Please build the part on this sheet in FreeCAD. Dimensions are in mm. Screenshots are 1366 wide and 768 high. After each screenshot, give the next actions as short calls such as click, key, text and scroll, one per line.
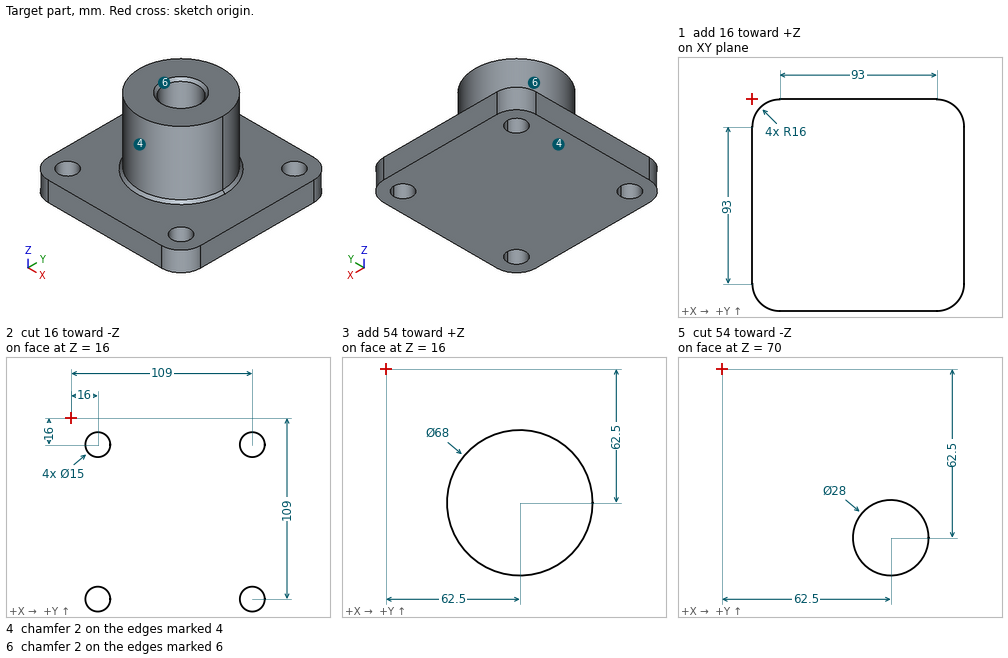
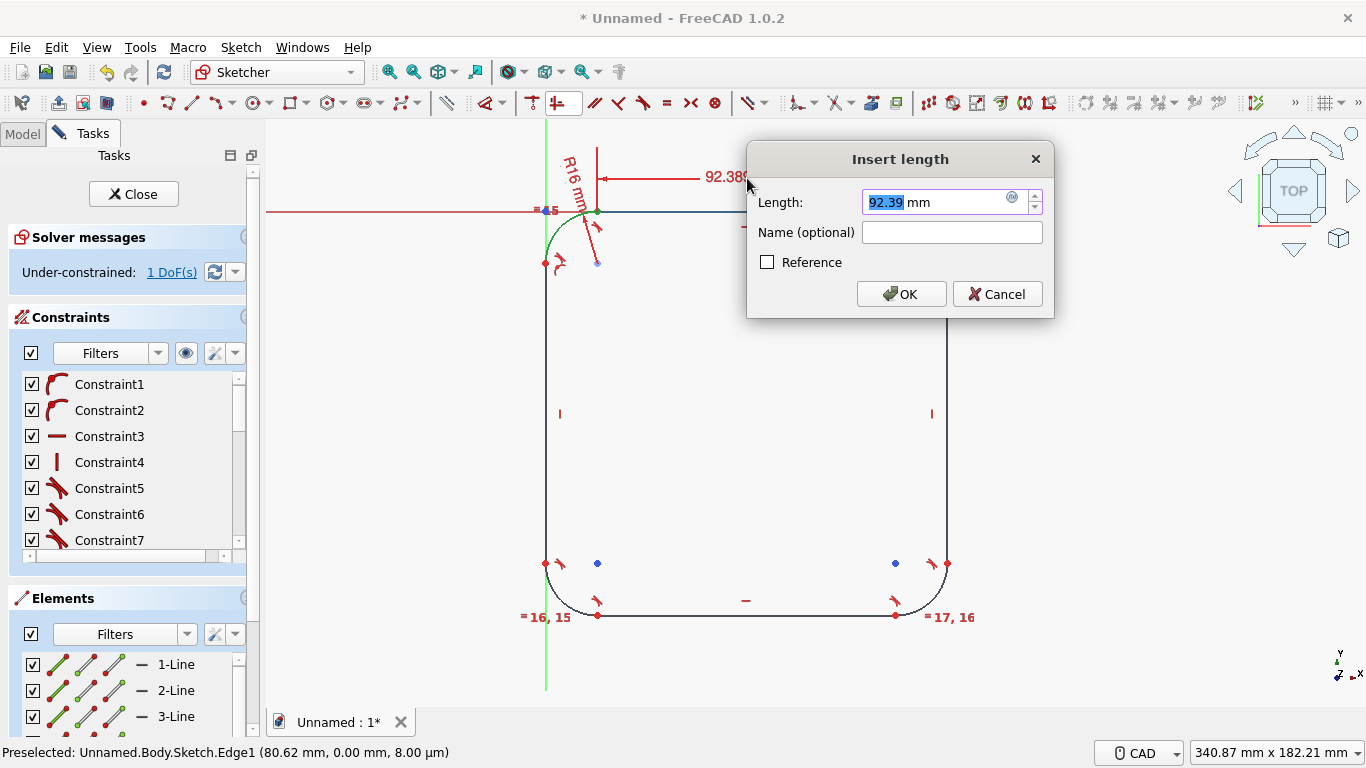
text(93)
key(Return)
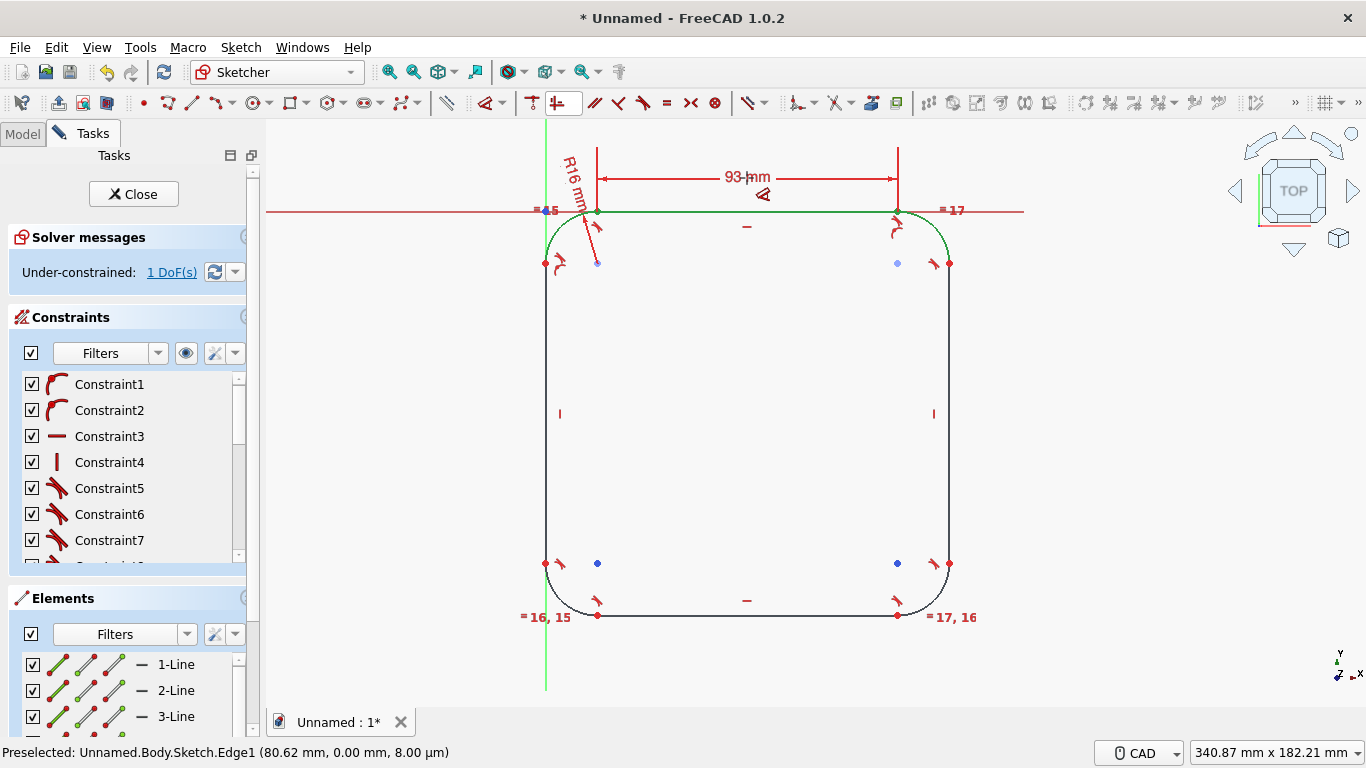
click(546, 353)
click(512, 414)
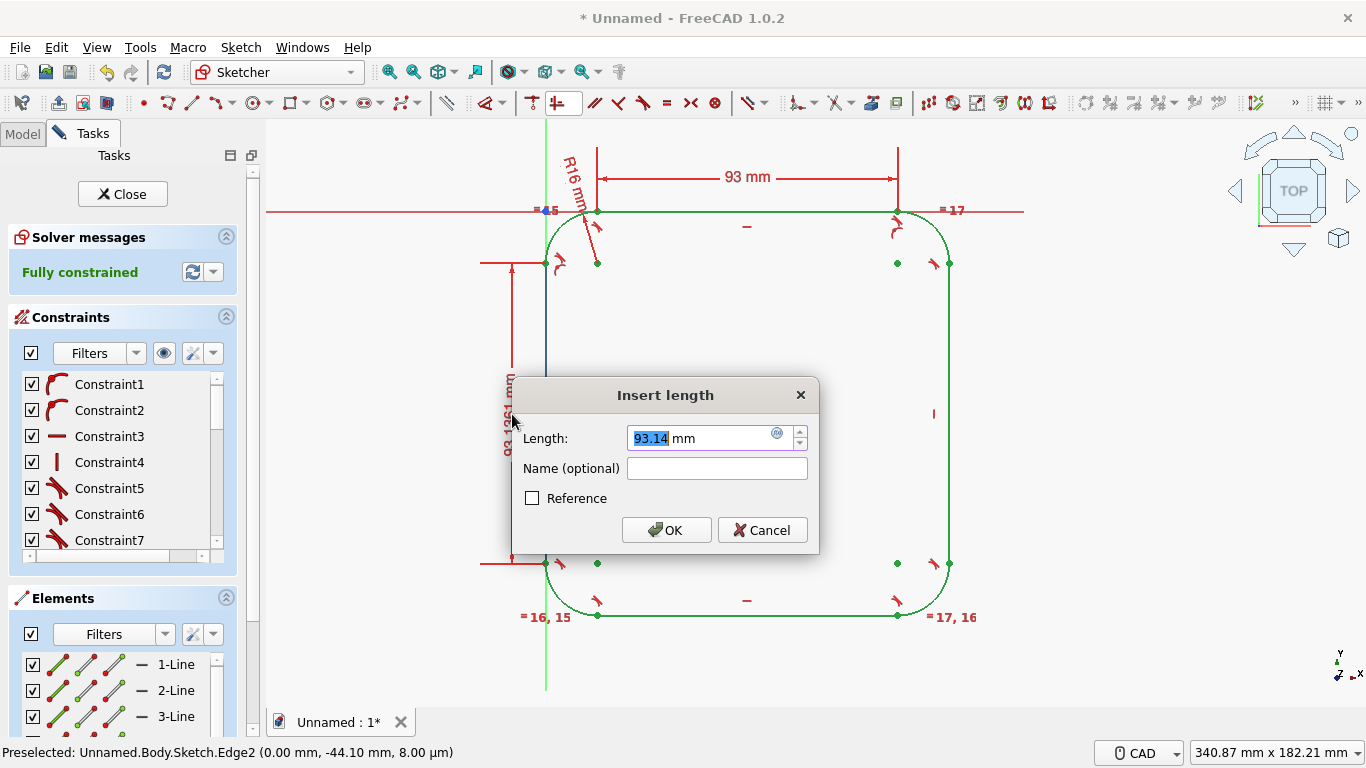
text(93)
key(Return)
key(Escape)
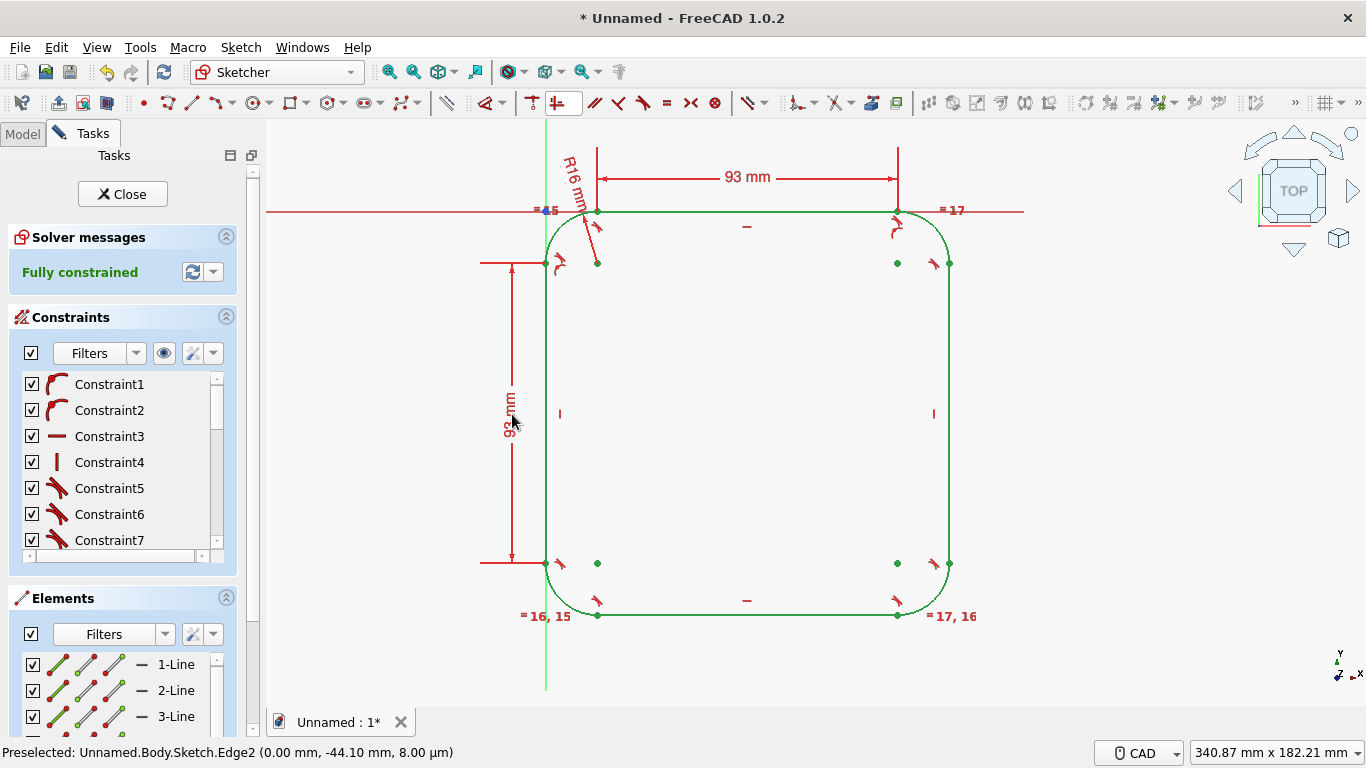
click(123, 194)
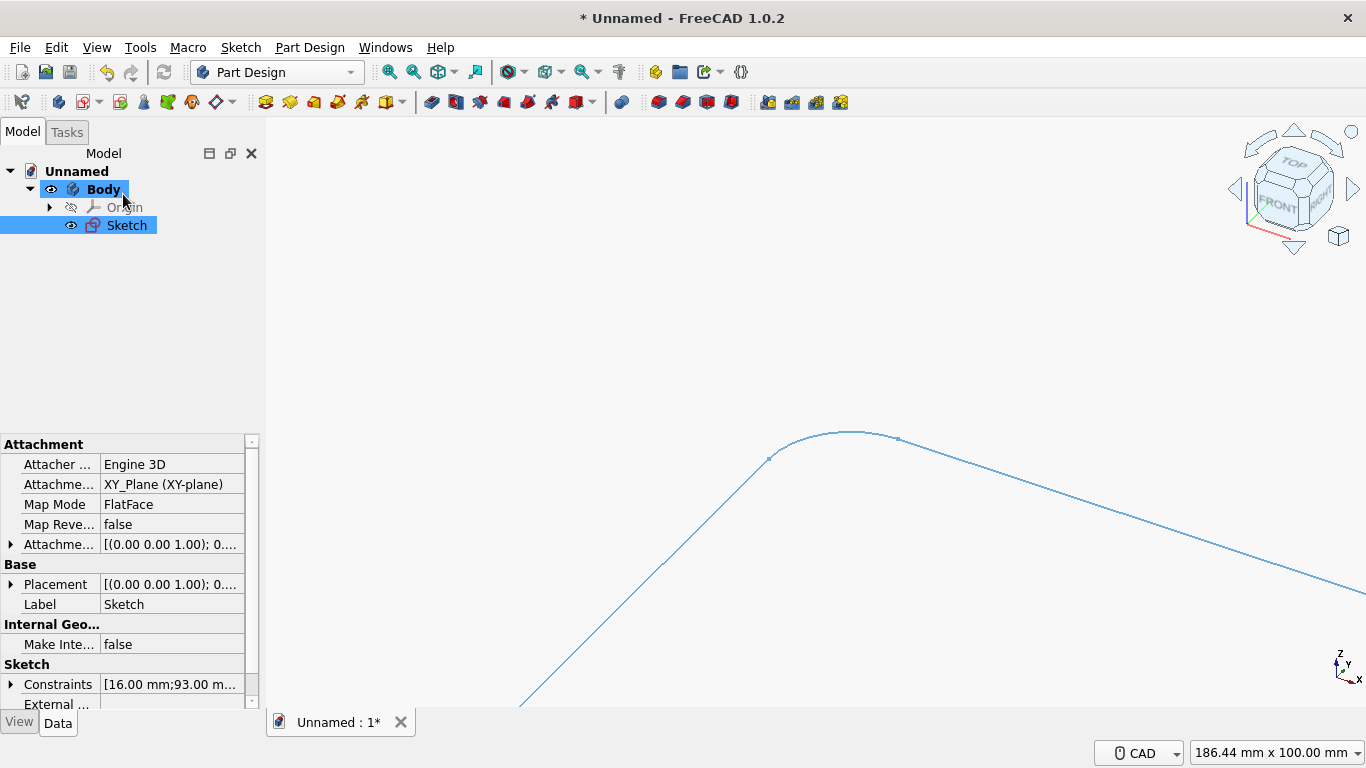
click(266, 102)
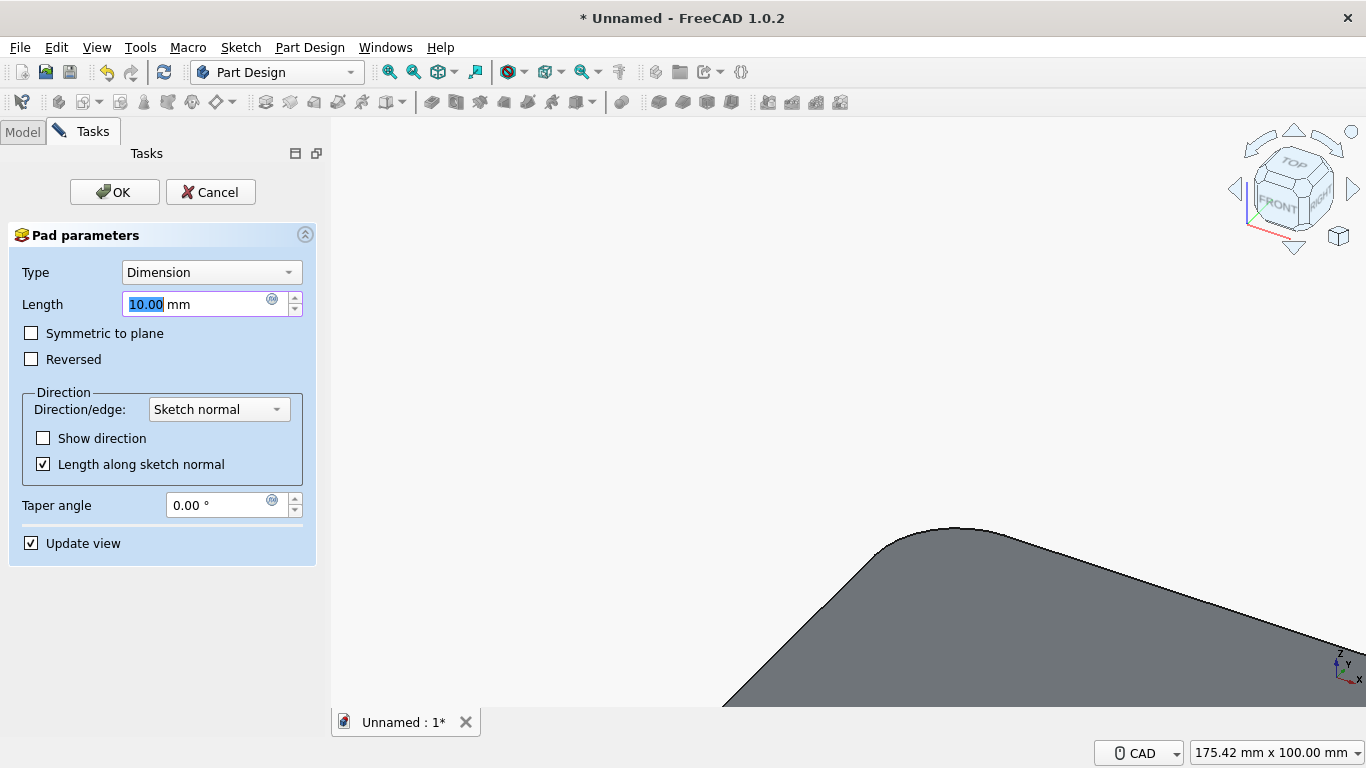
text(16)
key(Tab)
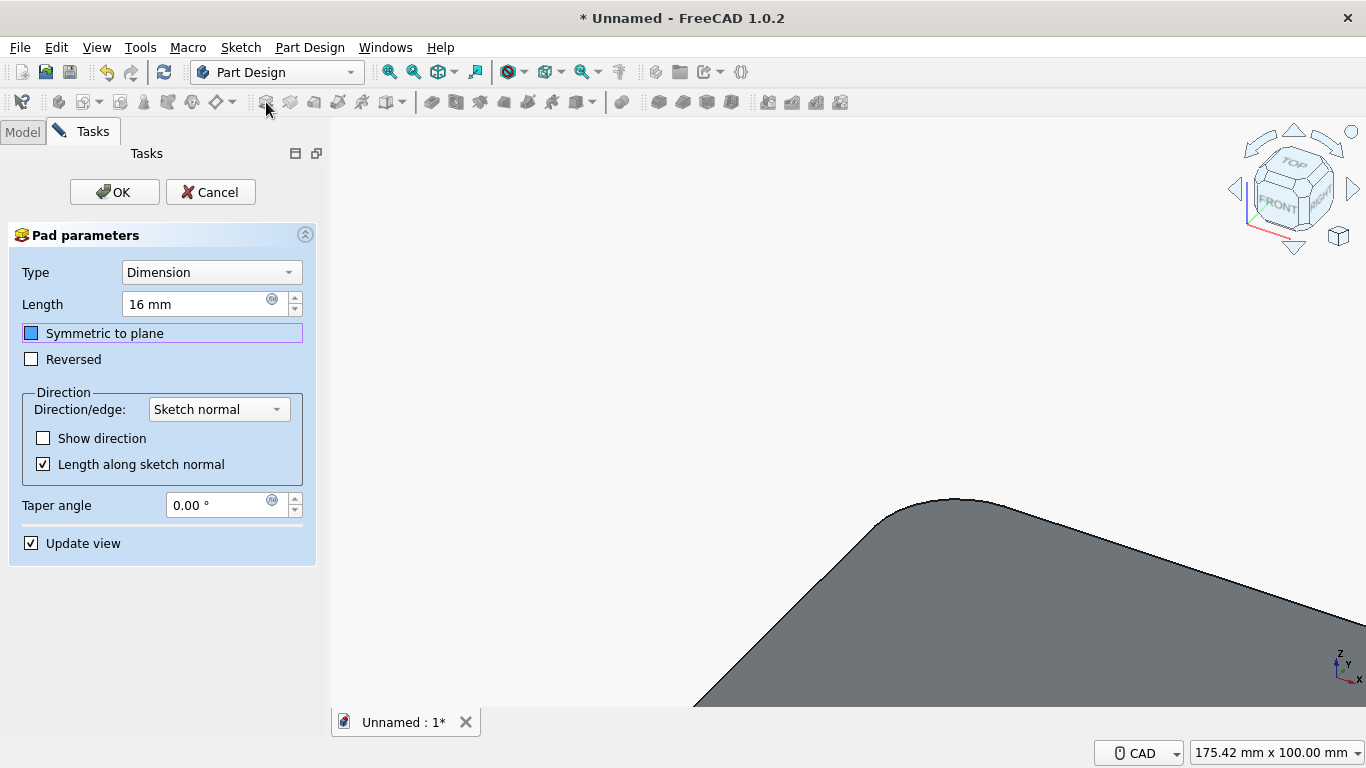
click(115, 192)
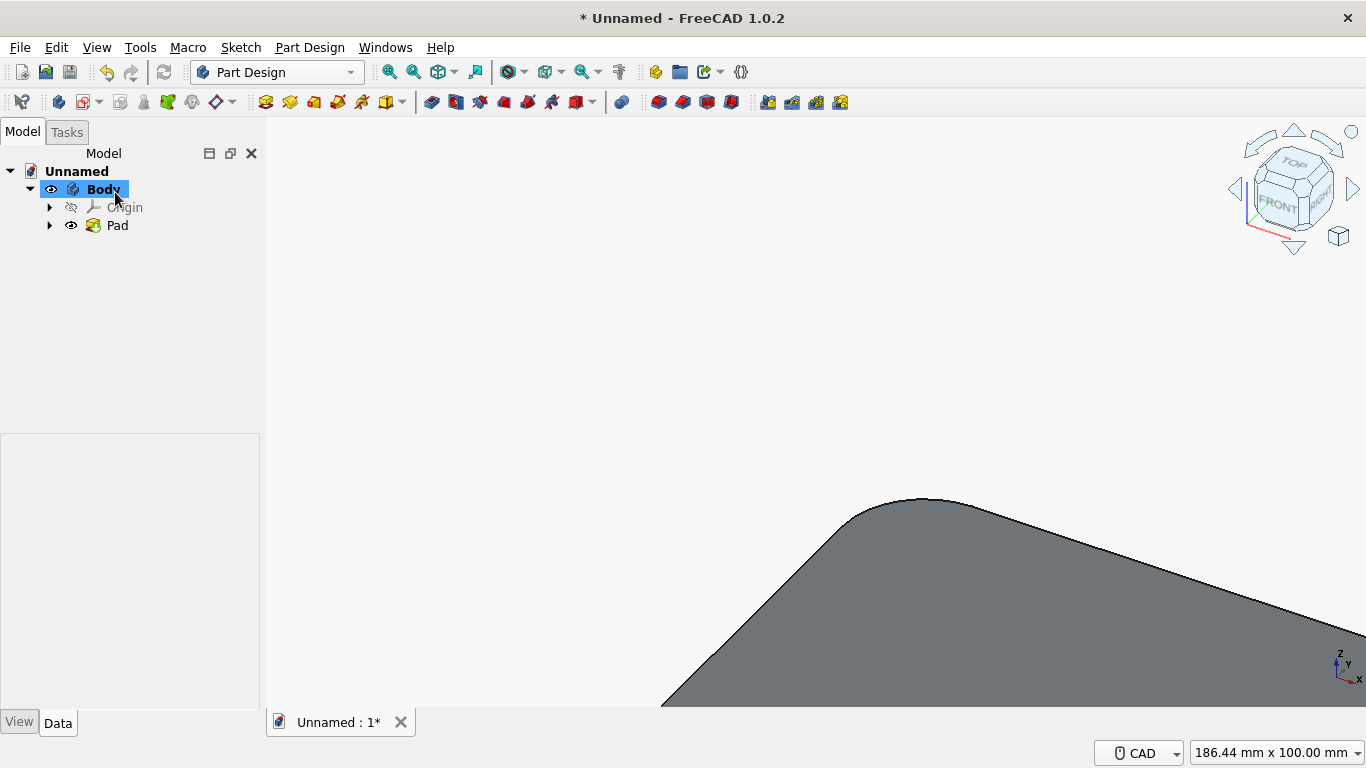
key(v)
key(f)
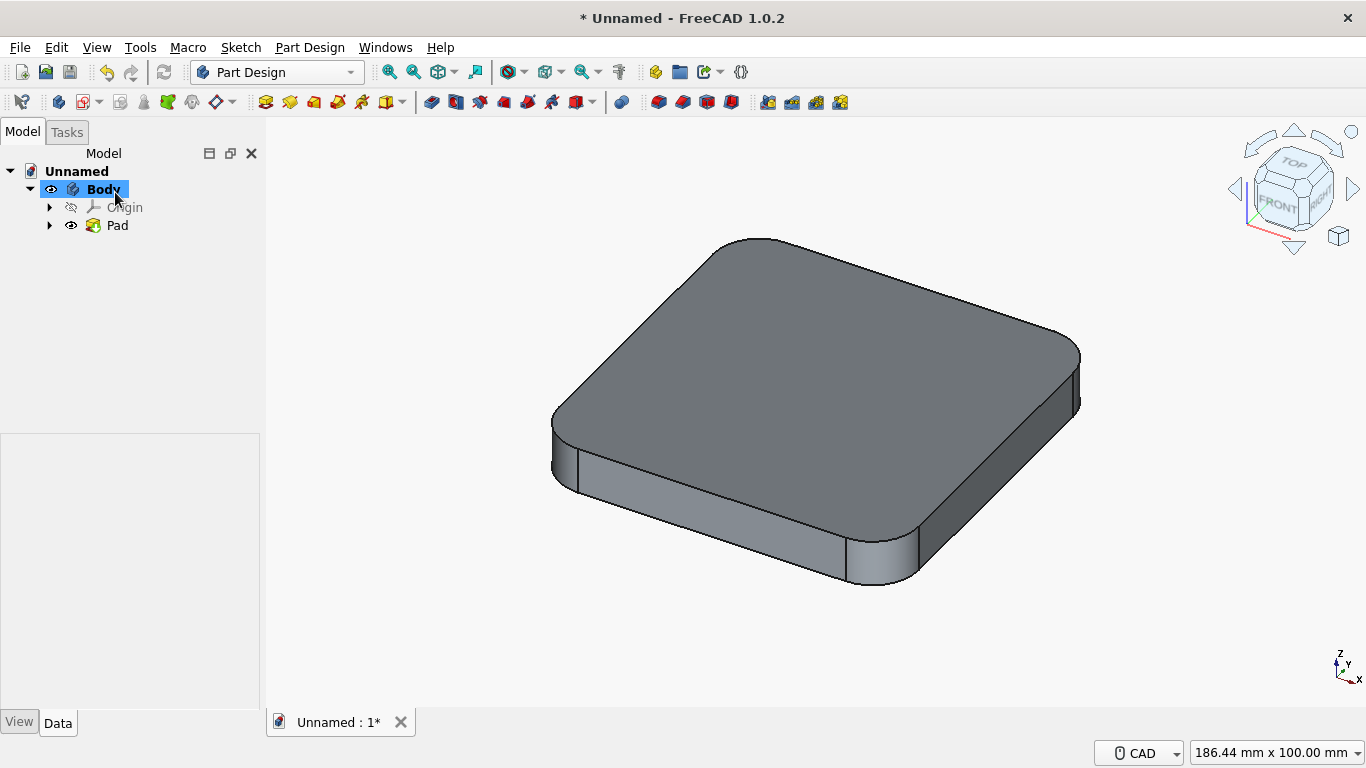
click(816, 389)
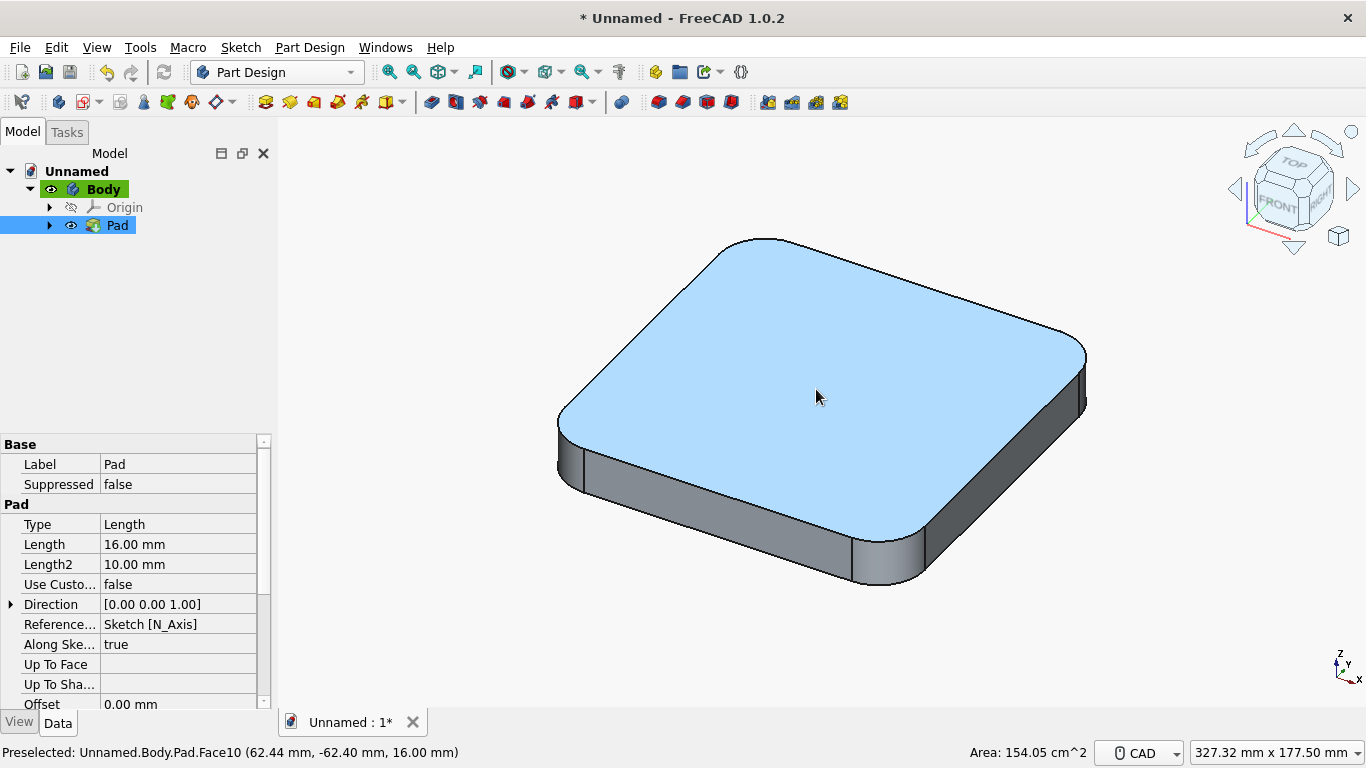
click(84, 102)